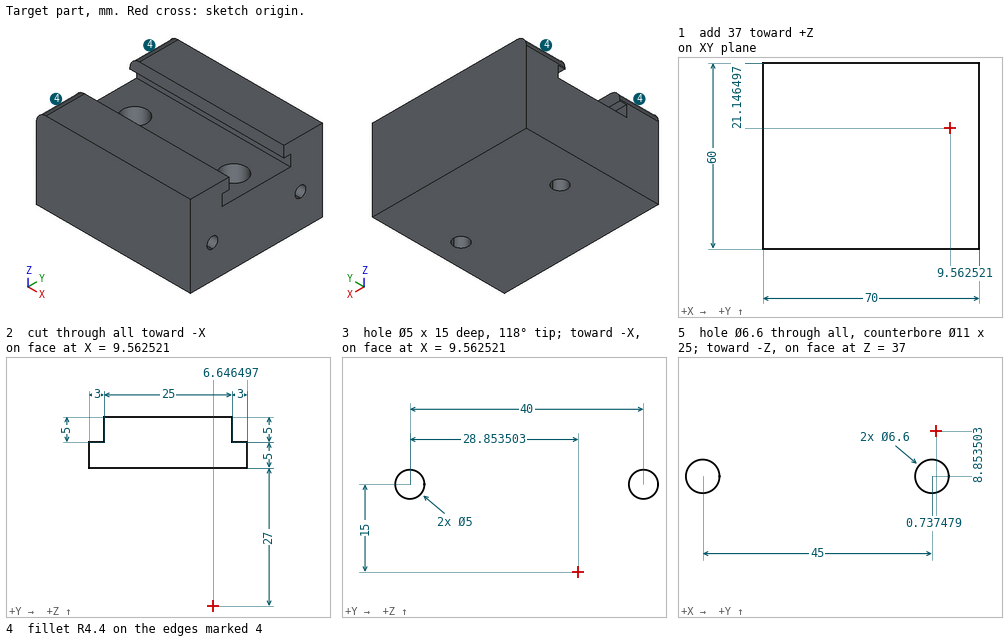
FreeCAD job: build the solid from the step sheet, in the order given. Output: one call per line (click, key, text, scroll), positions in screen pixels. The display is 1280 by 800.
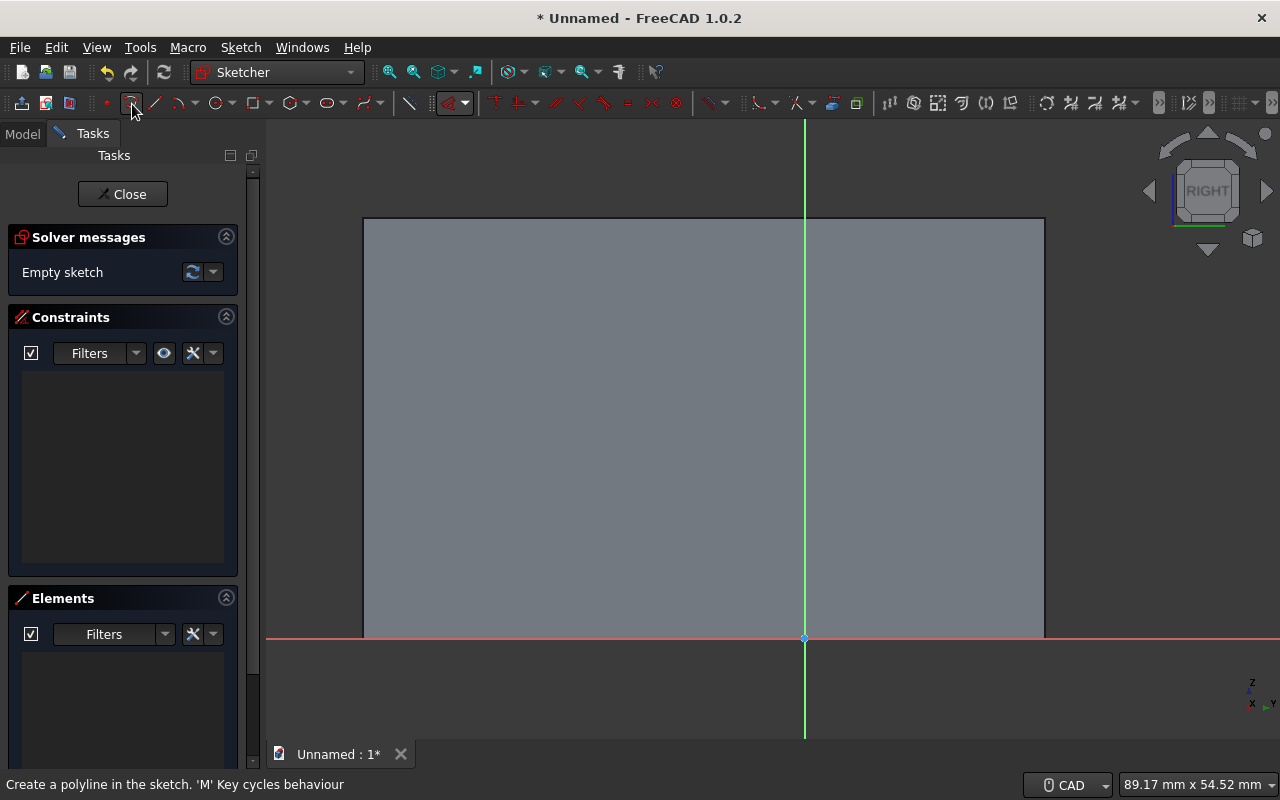
click(881, 332)
click(881, 275)
click(846, 275)
click(846, 218)
click(562, 218)
click(562, 275)
click(528, 275)
click(528, 332)
click(881, 333)
key(Escape)
key(Escape)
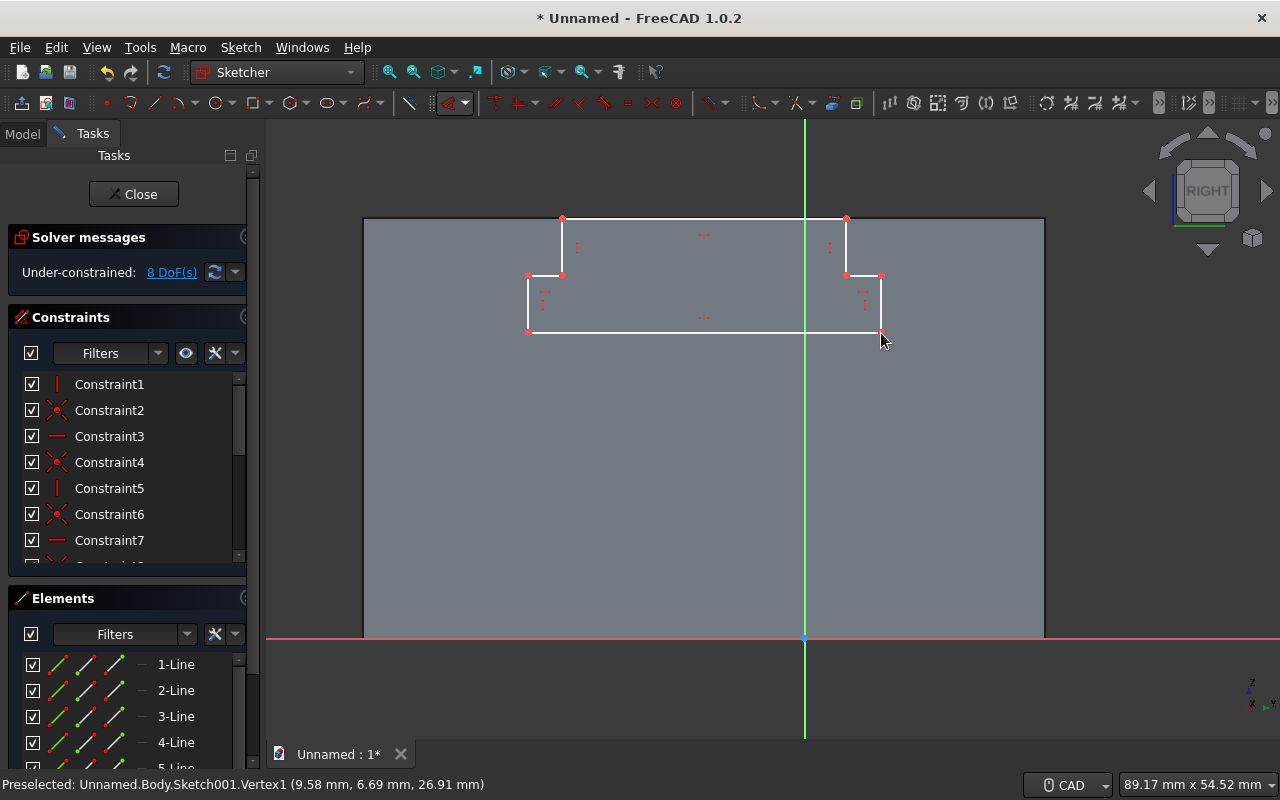
click(881, 316)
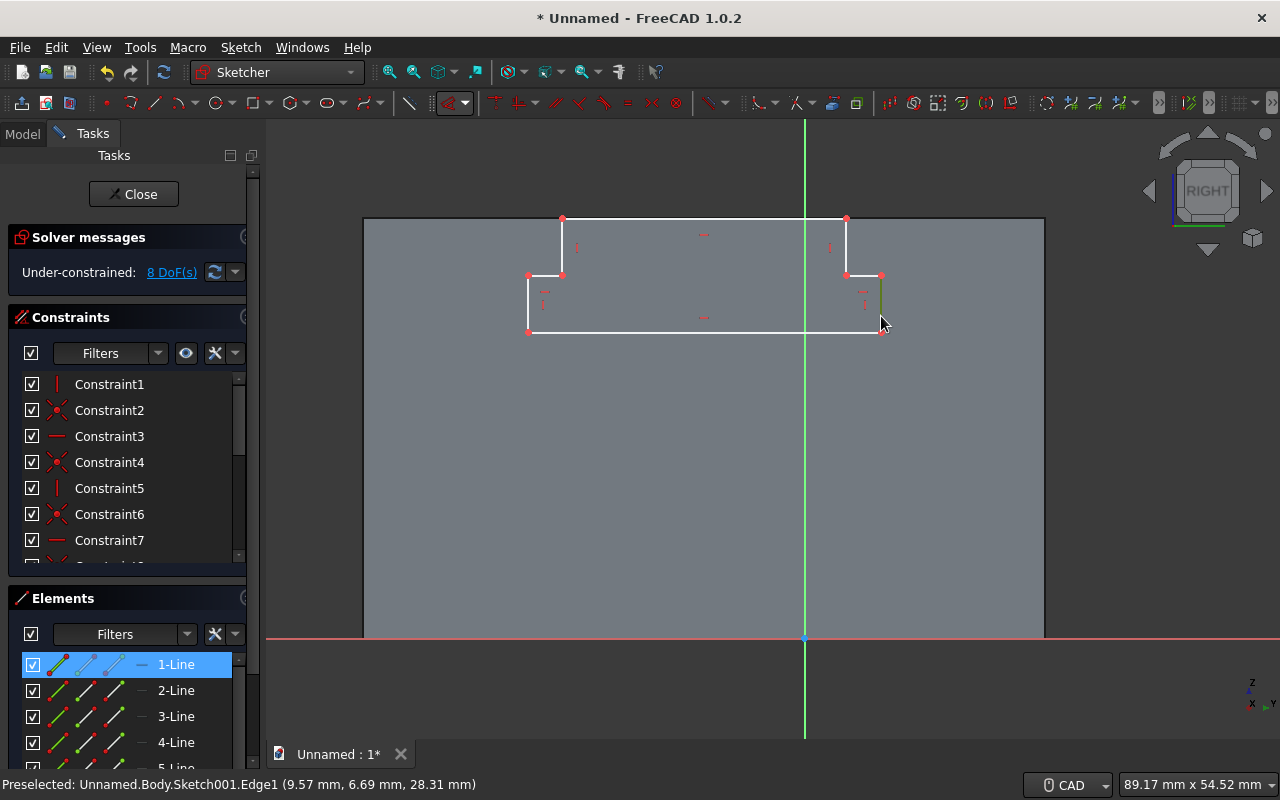
key(i)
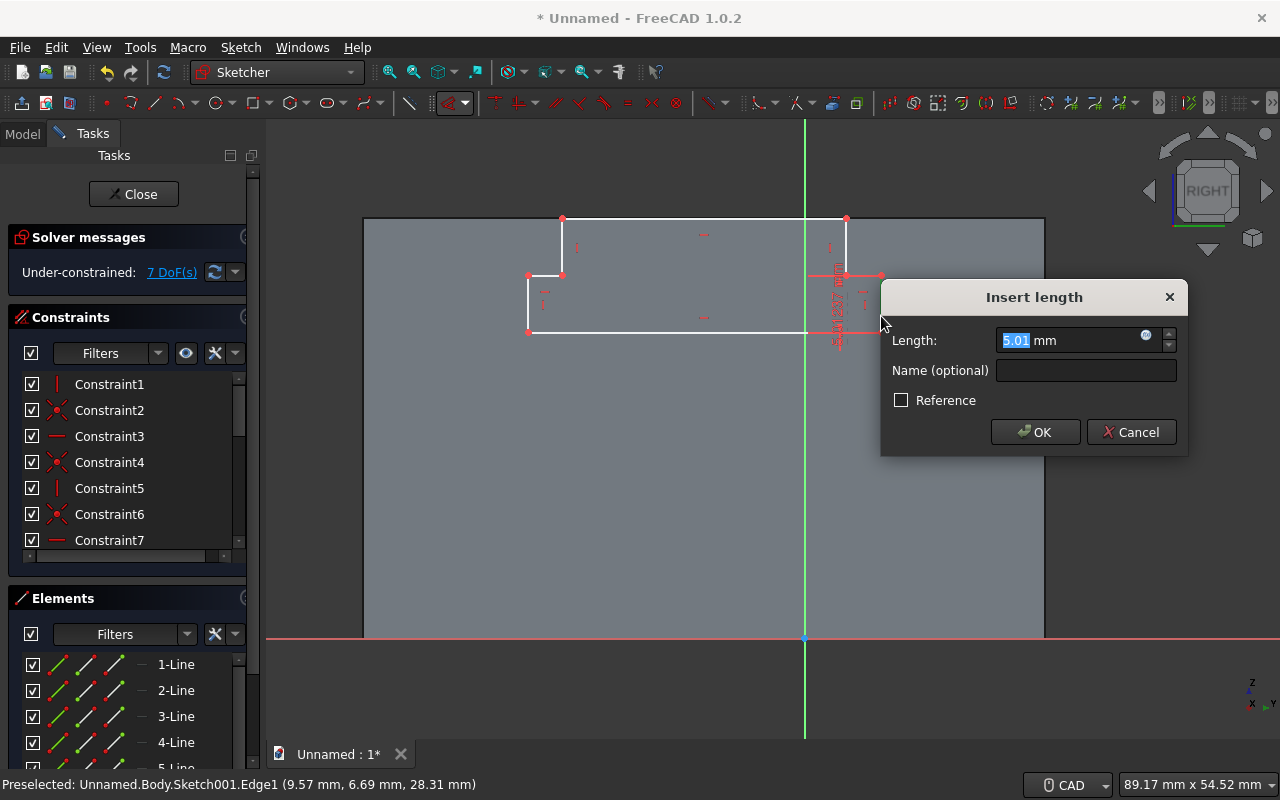
text(5)
key(Return)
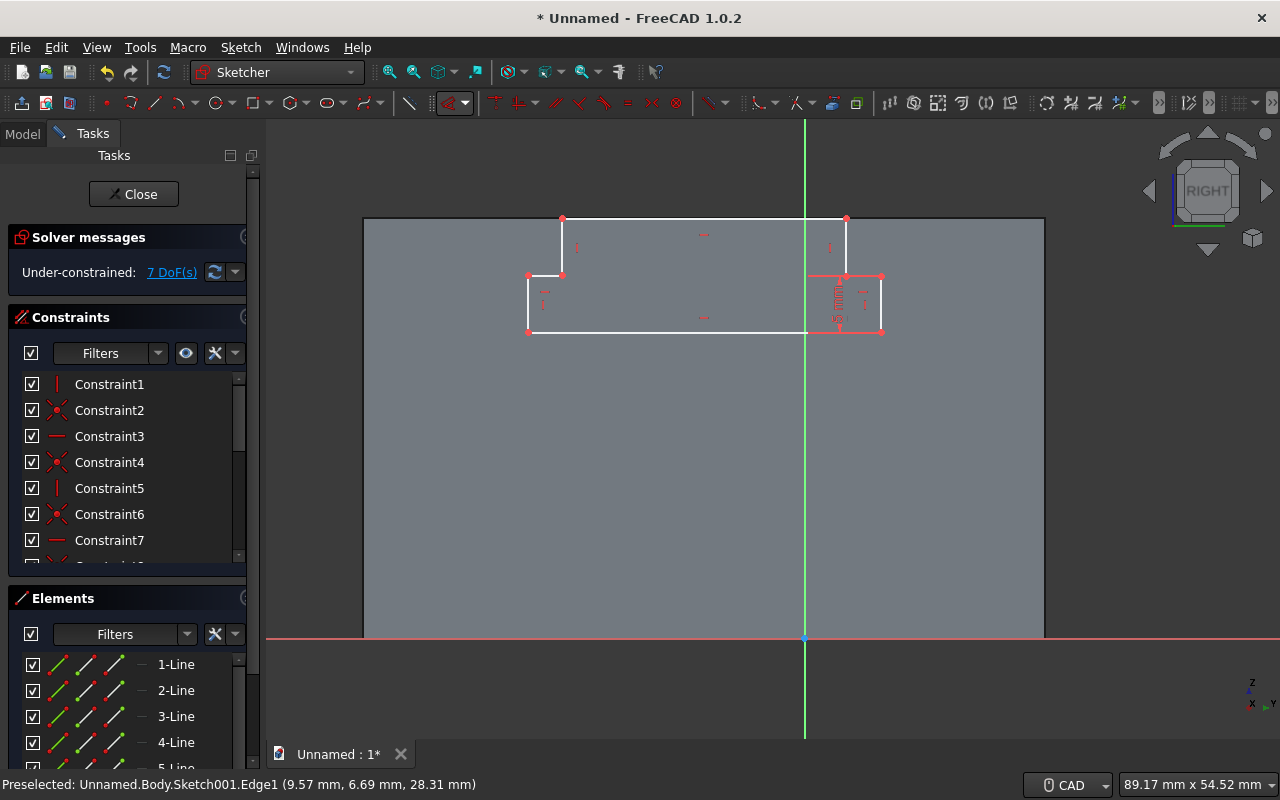
scroll(870, 276, up, 2)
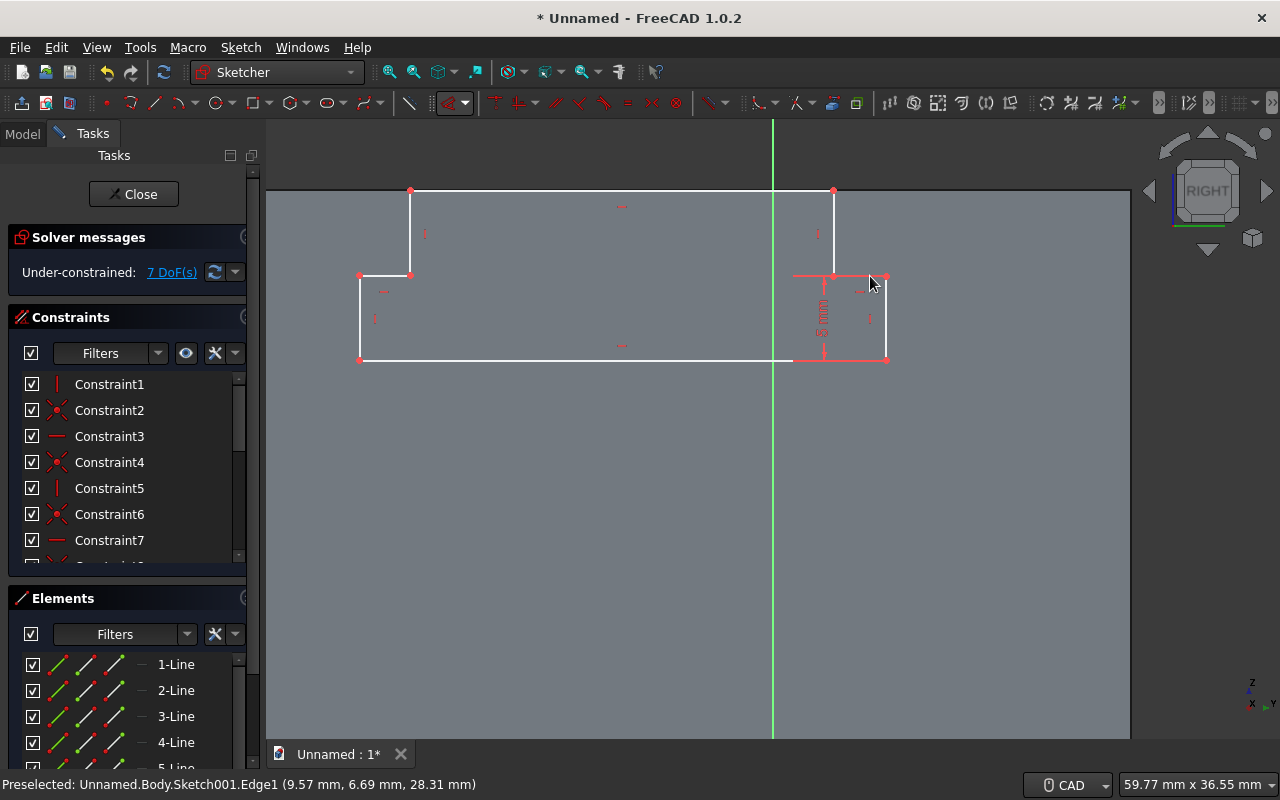
click(870, 276)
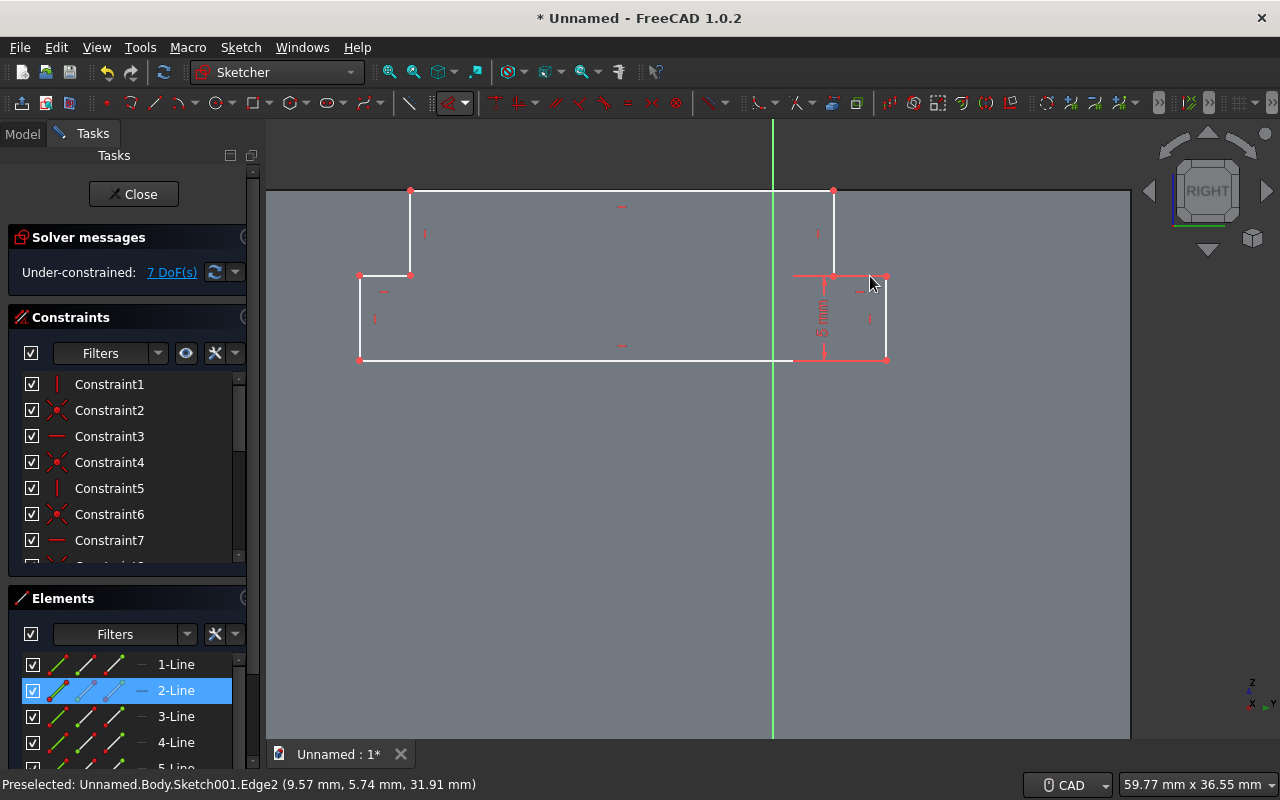
click(468, 104)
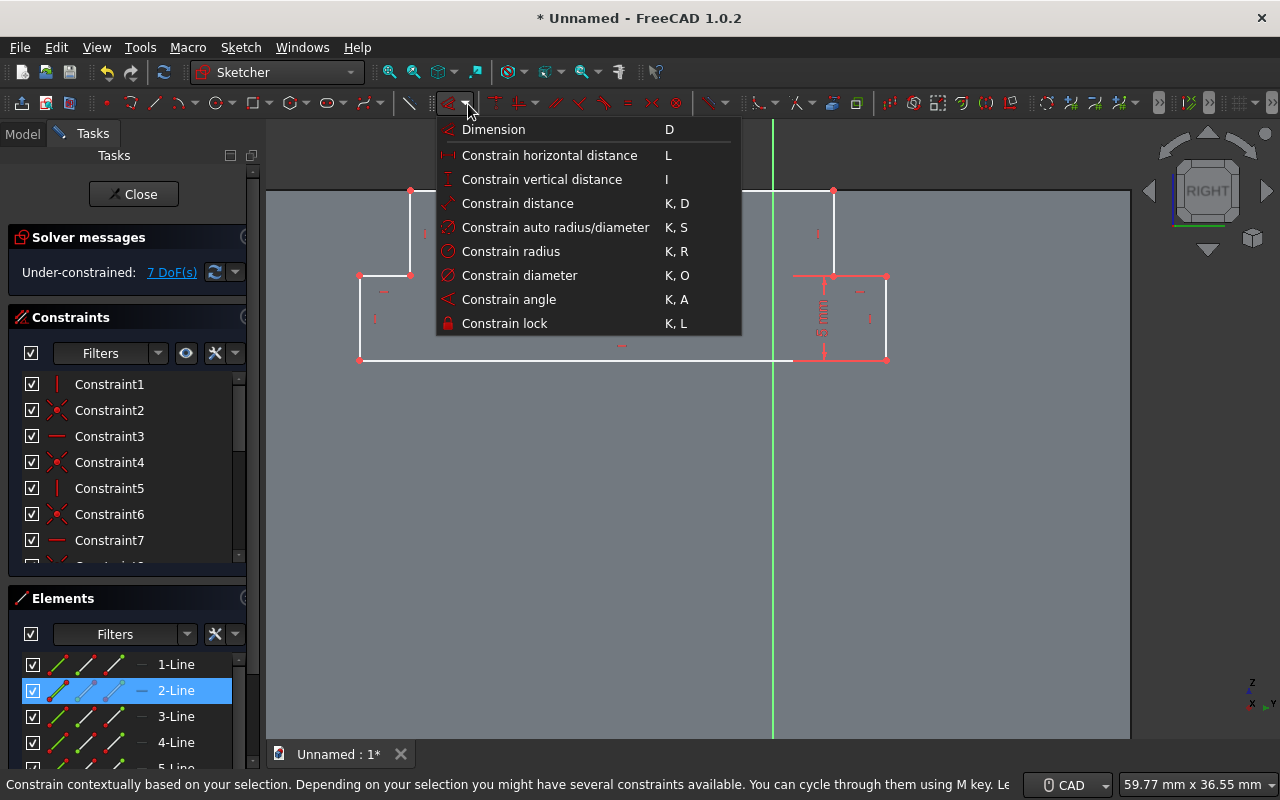
click(589, 155)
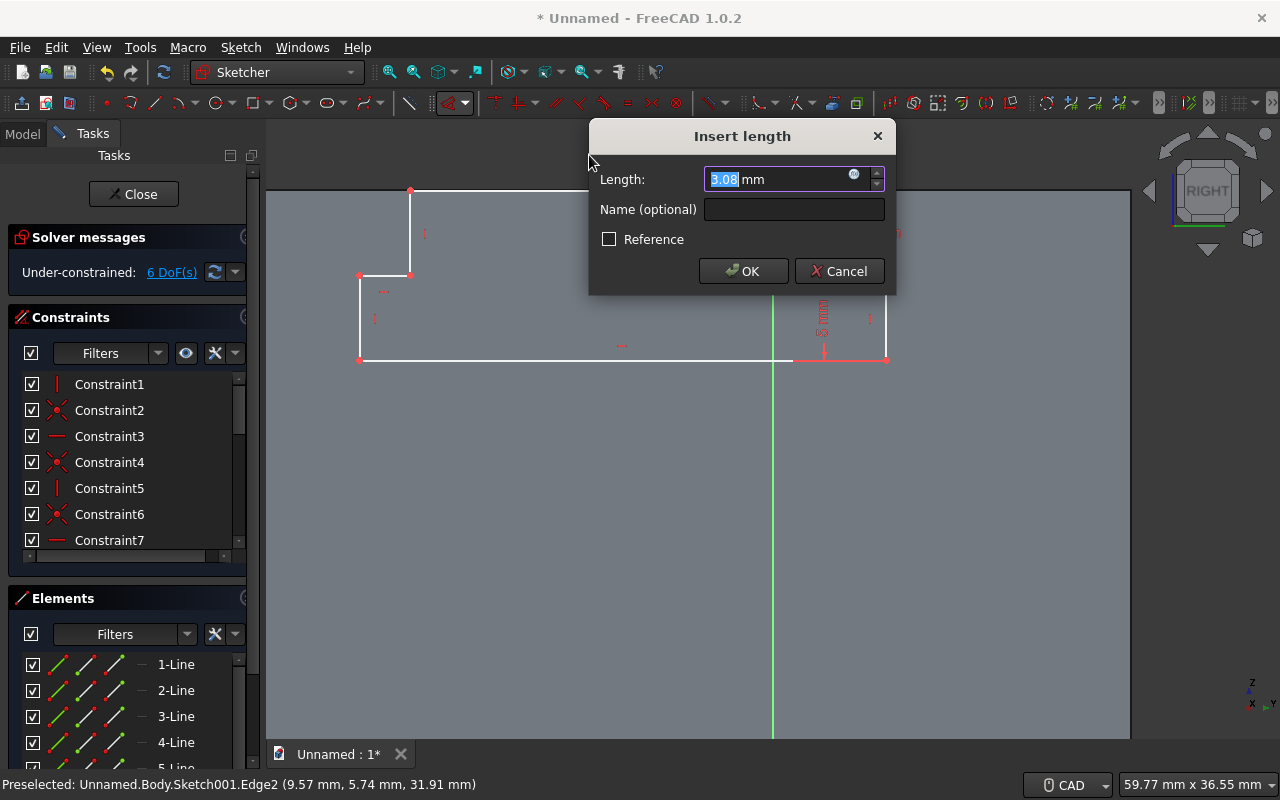
text(3)
key(Return)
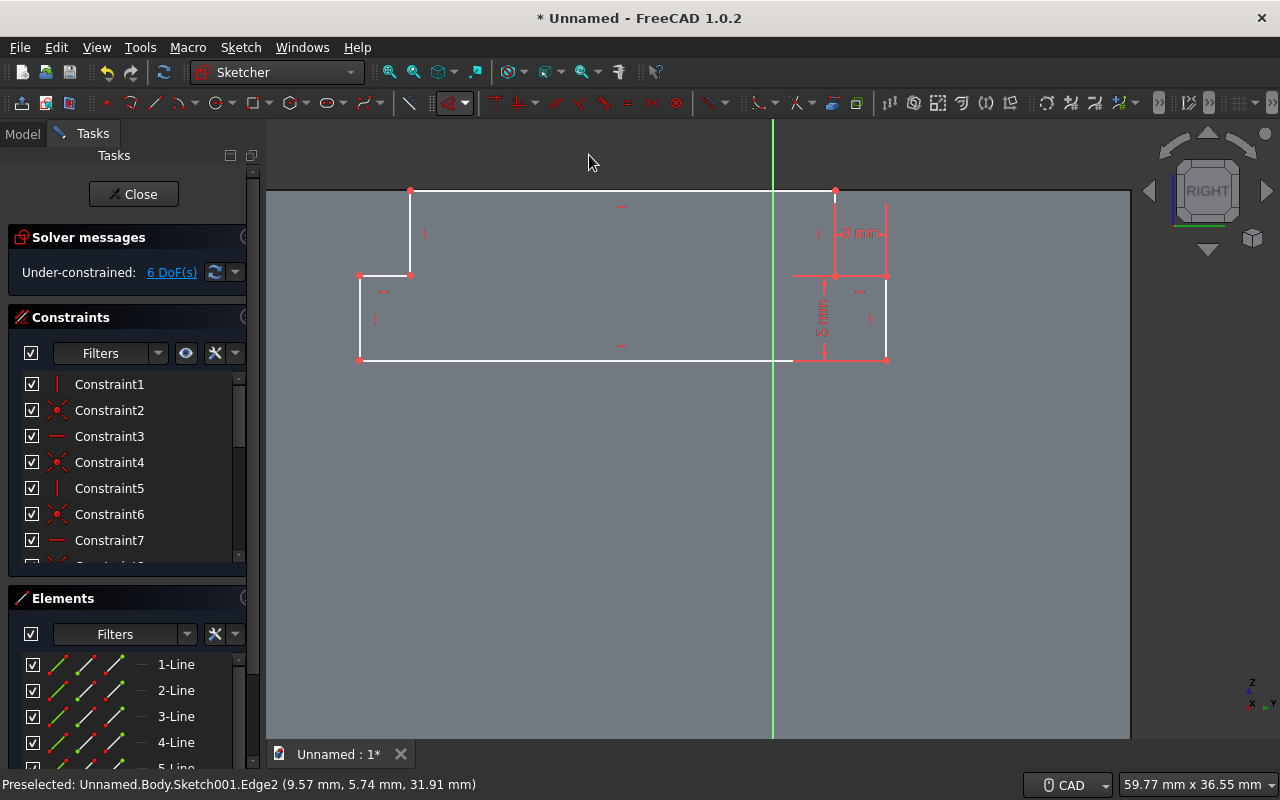
click(835, 251)